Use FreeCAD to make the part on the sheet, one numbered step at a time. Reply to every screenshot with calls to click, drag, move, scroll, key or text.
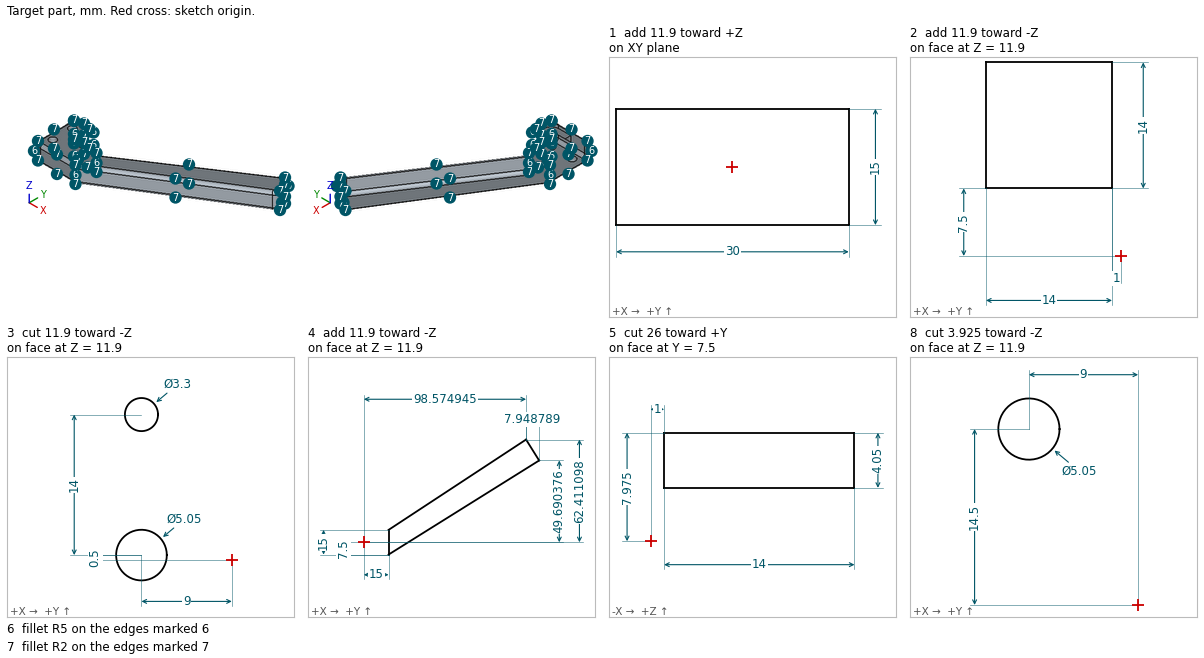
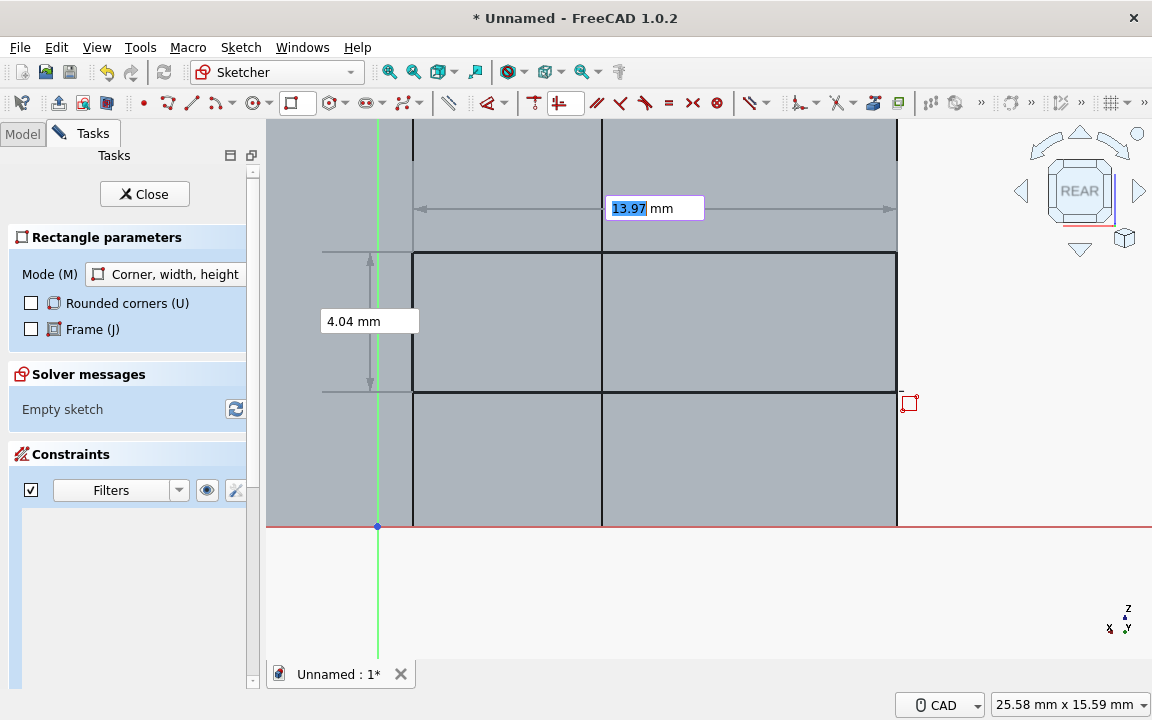
text(14)
key(Tab)
text(4.05)
key(Return)
key(Escape)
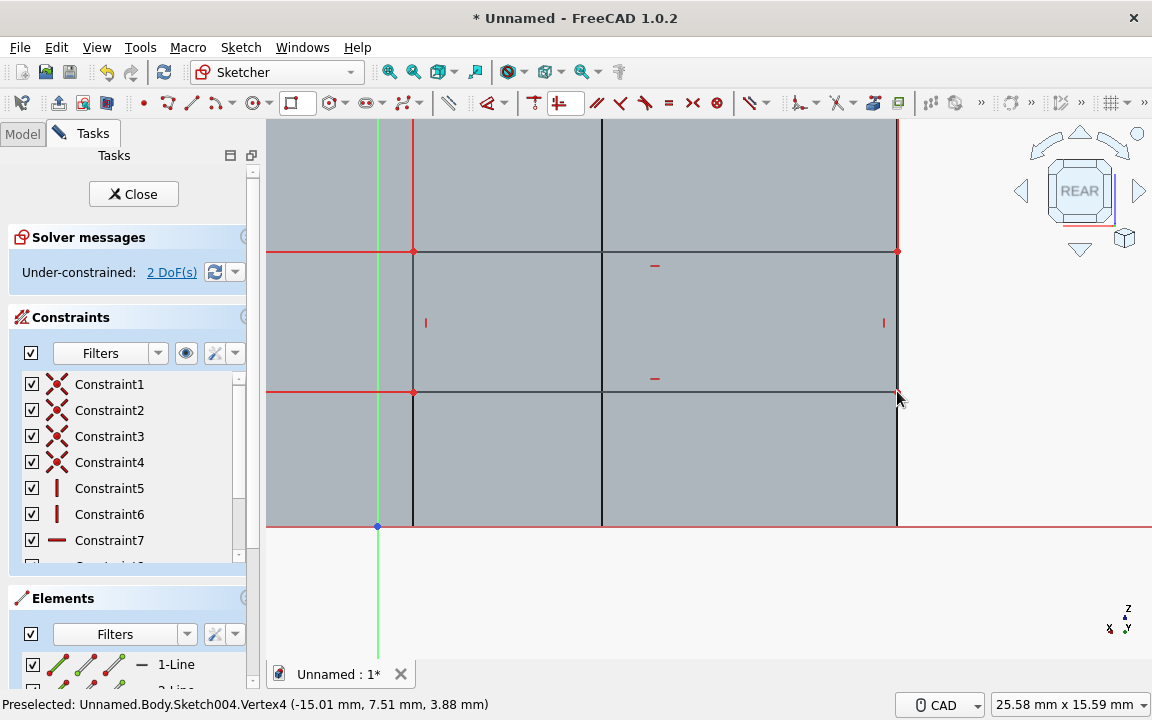
key(d)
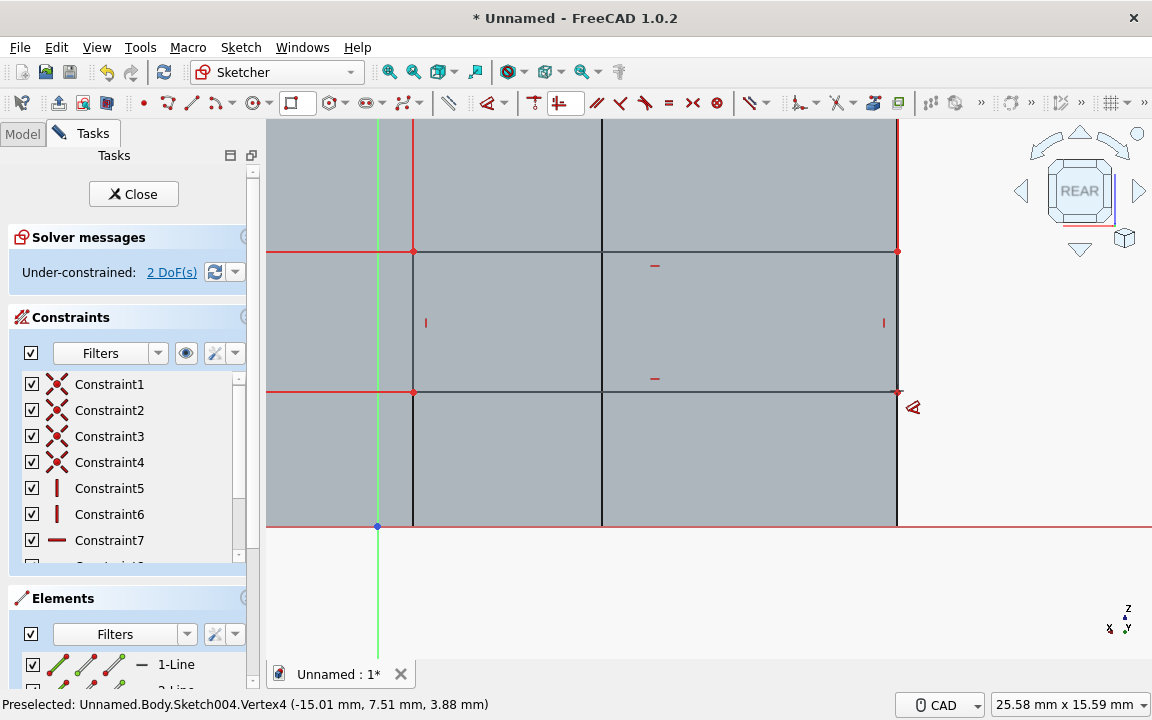
click(413, 252)
click(395, 561)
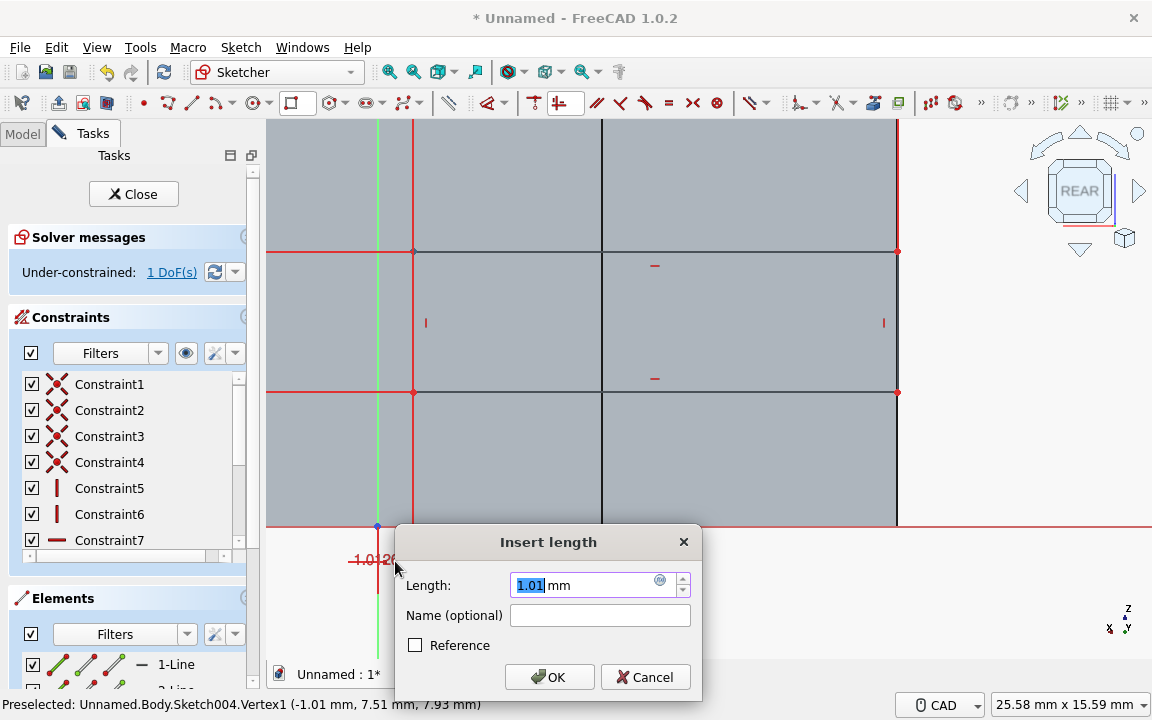
text(1)
key(Return)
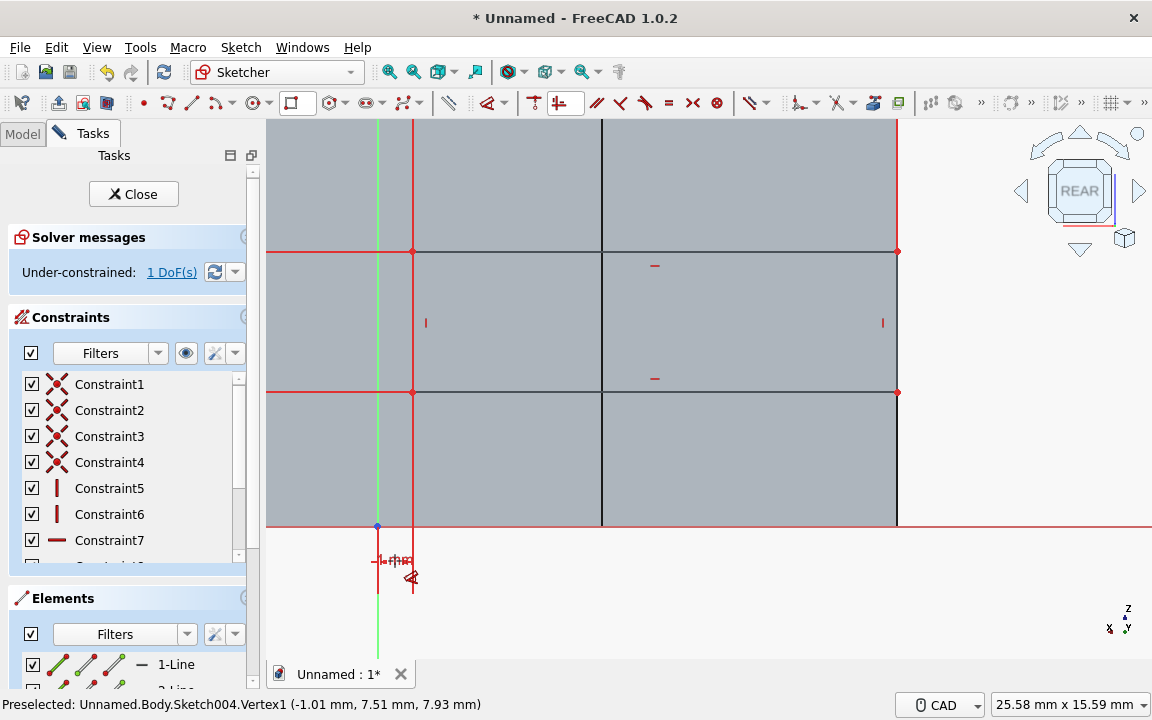
click(413, 252)
click(344, 389)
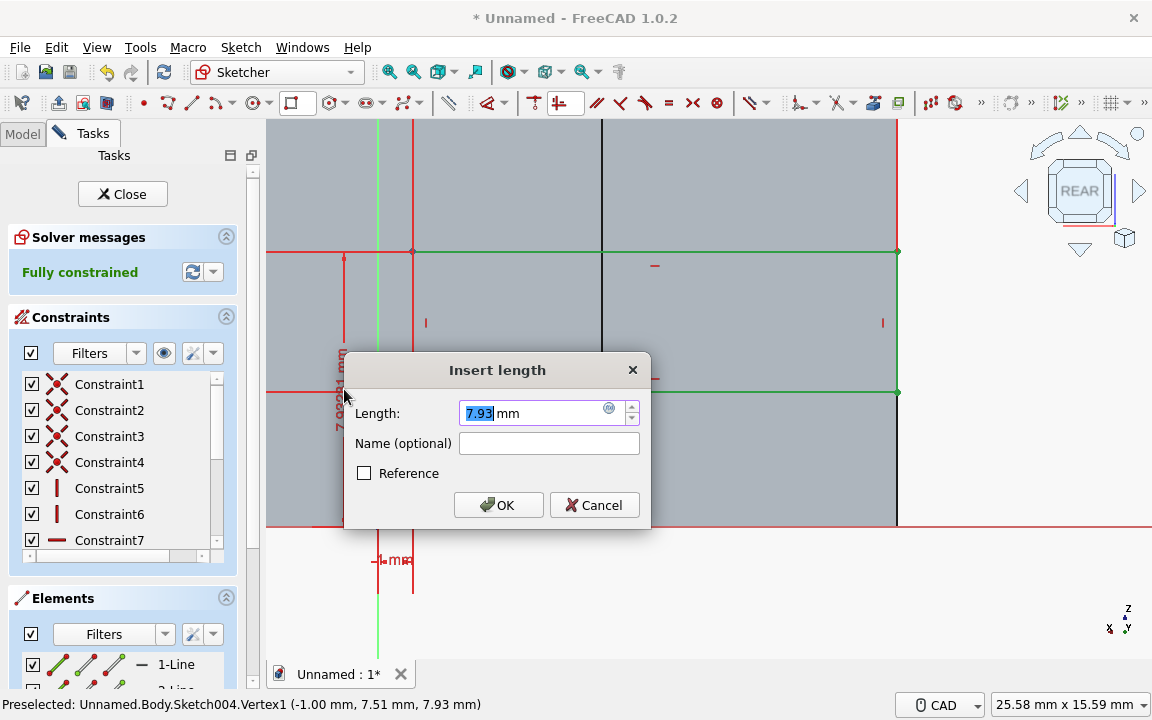
text(7.975)
key(Return)
key(Escape)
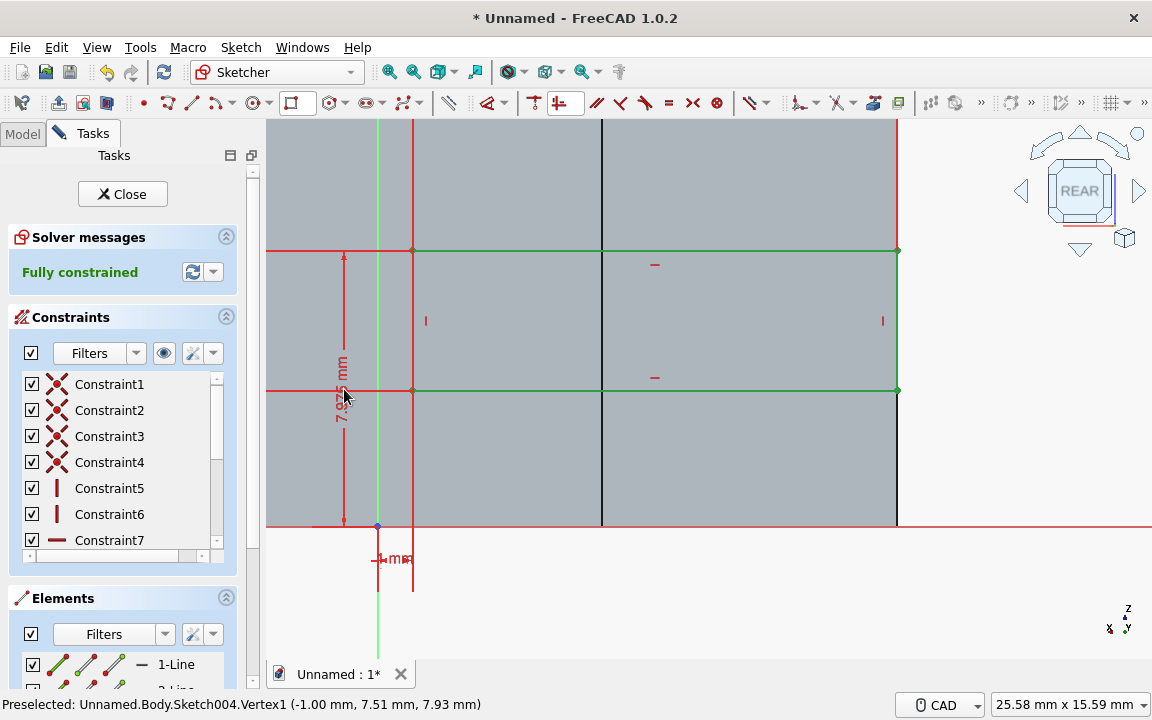
click(123, 194)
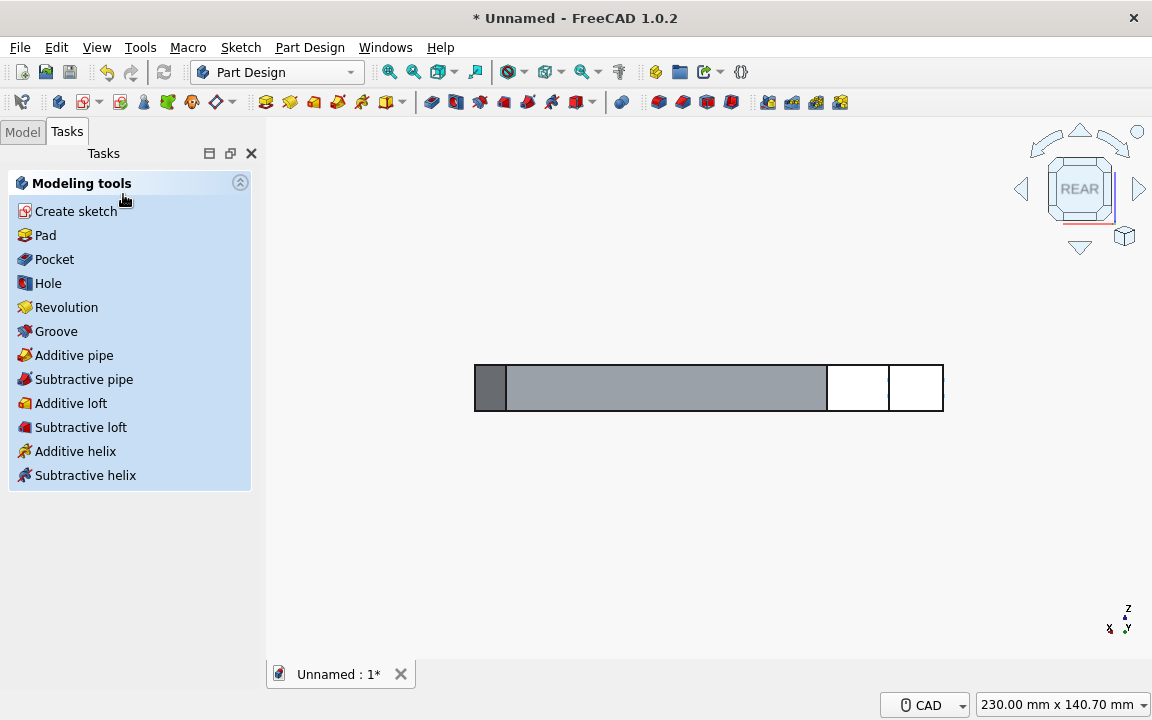
click(432, 102)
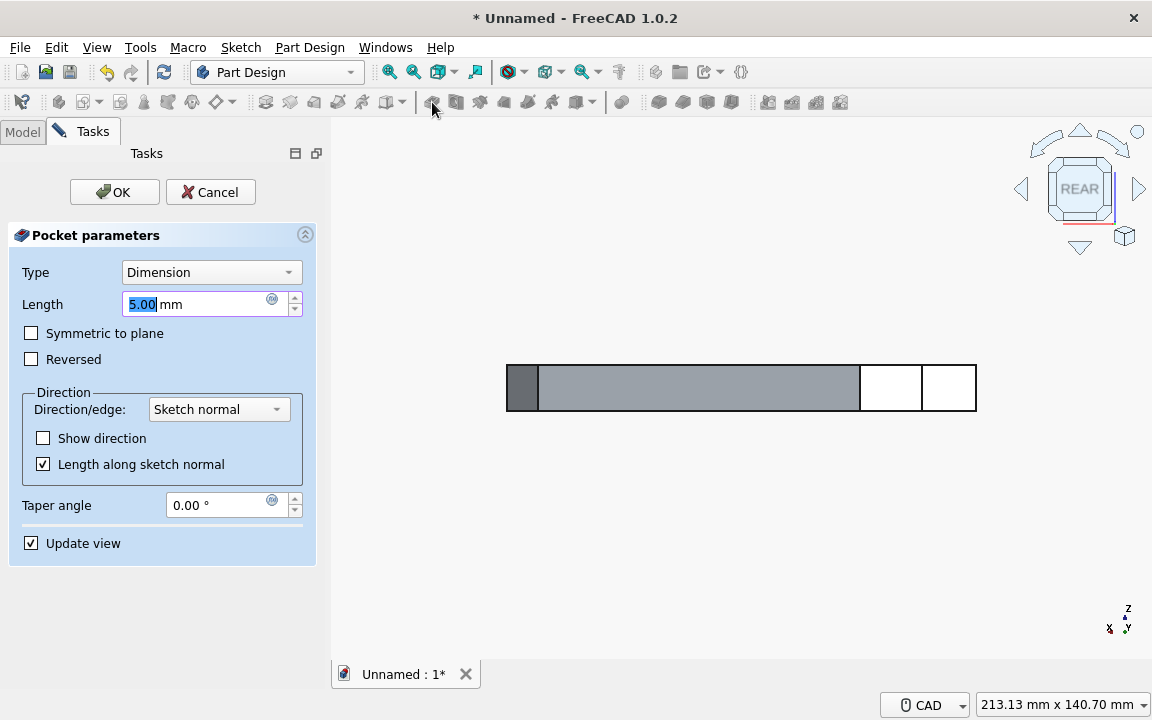
text(26)
key(Tab)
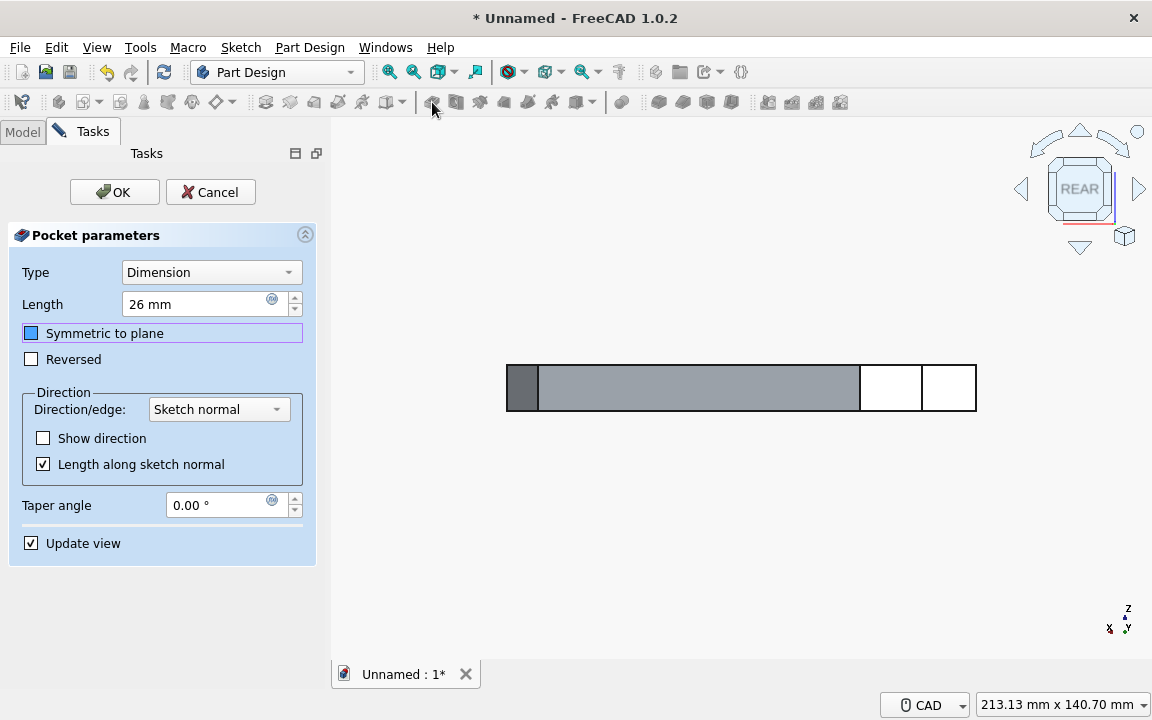
click(30, 359)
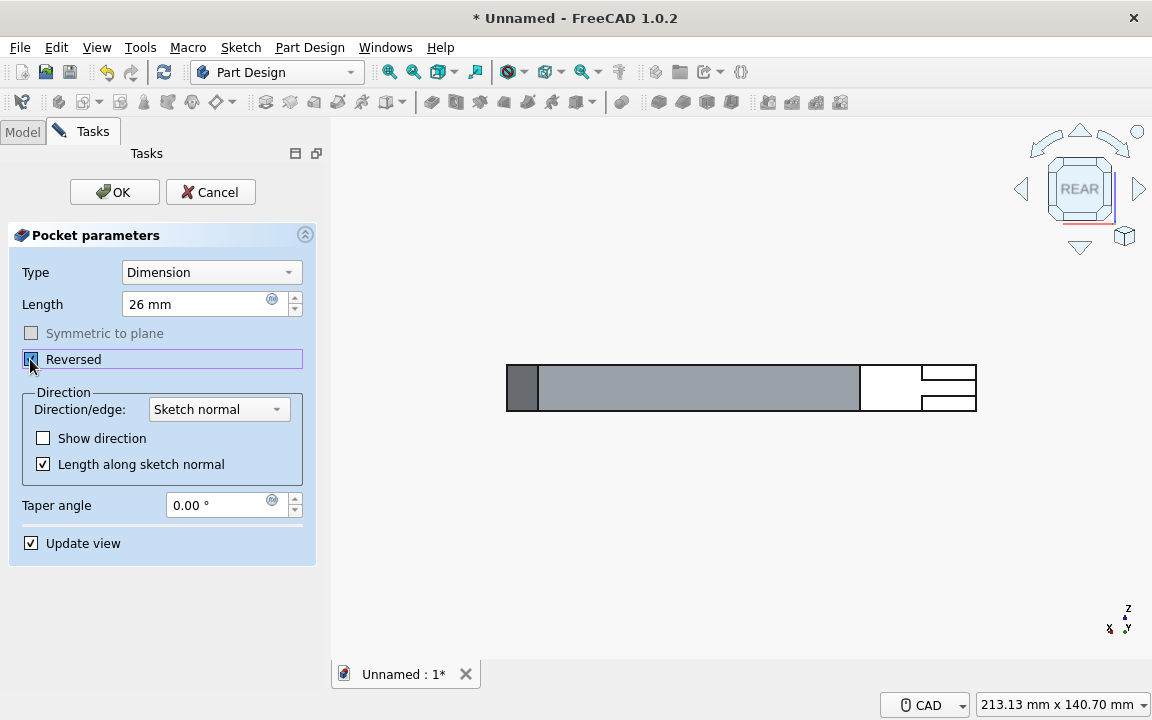
click(115, 192)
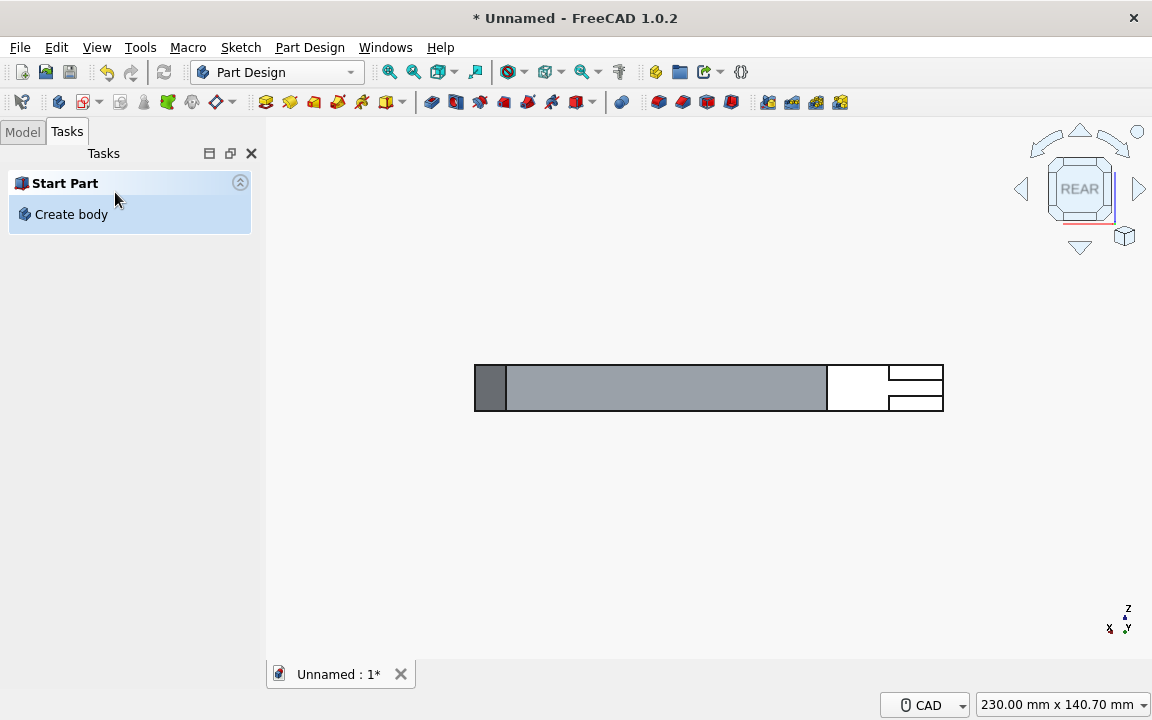
click(943, 402)